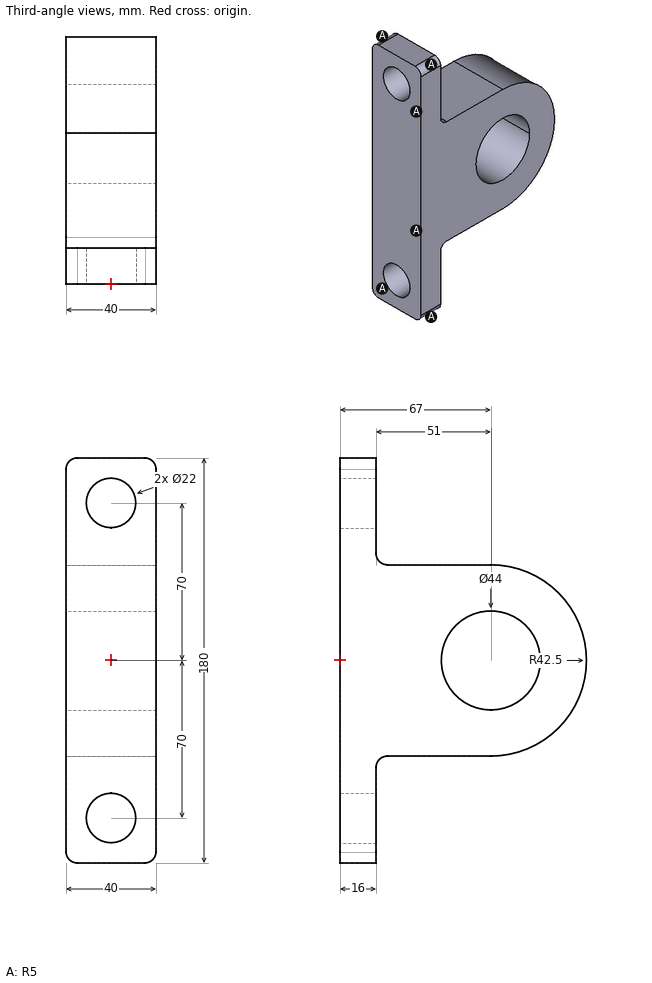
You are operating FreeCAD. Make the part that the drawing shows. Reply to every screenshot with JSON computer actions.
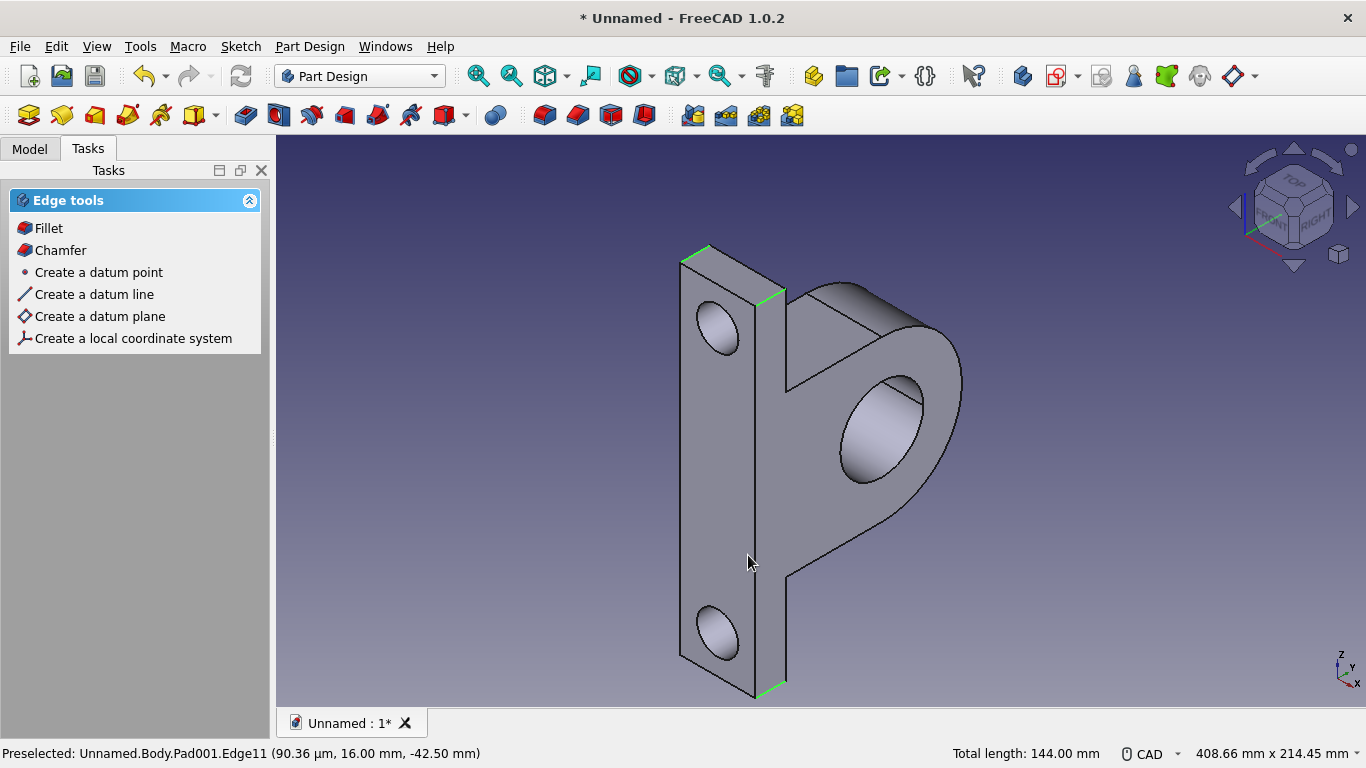
{"action": "left_click", "coordinate": [545, 116]}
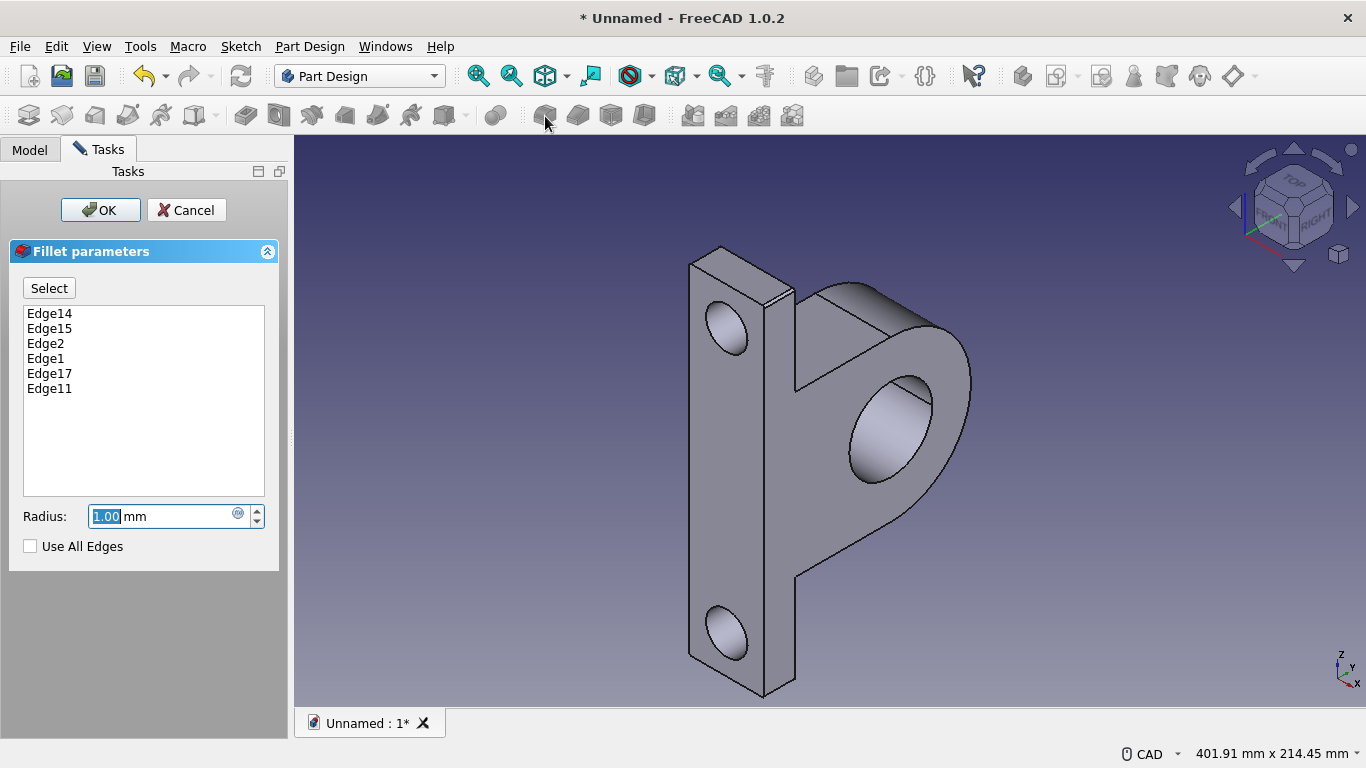
{"action": "type", "text": "5"}
{"action": "key", "text": "Tab"}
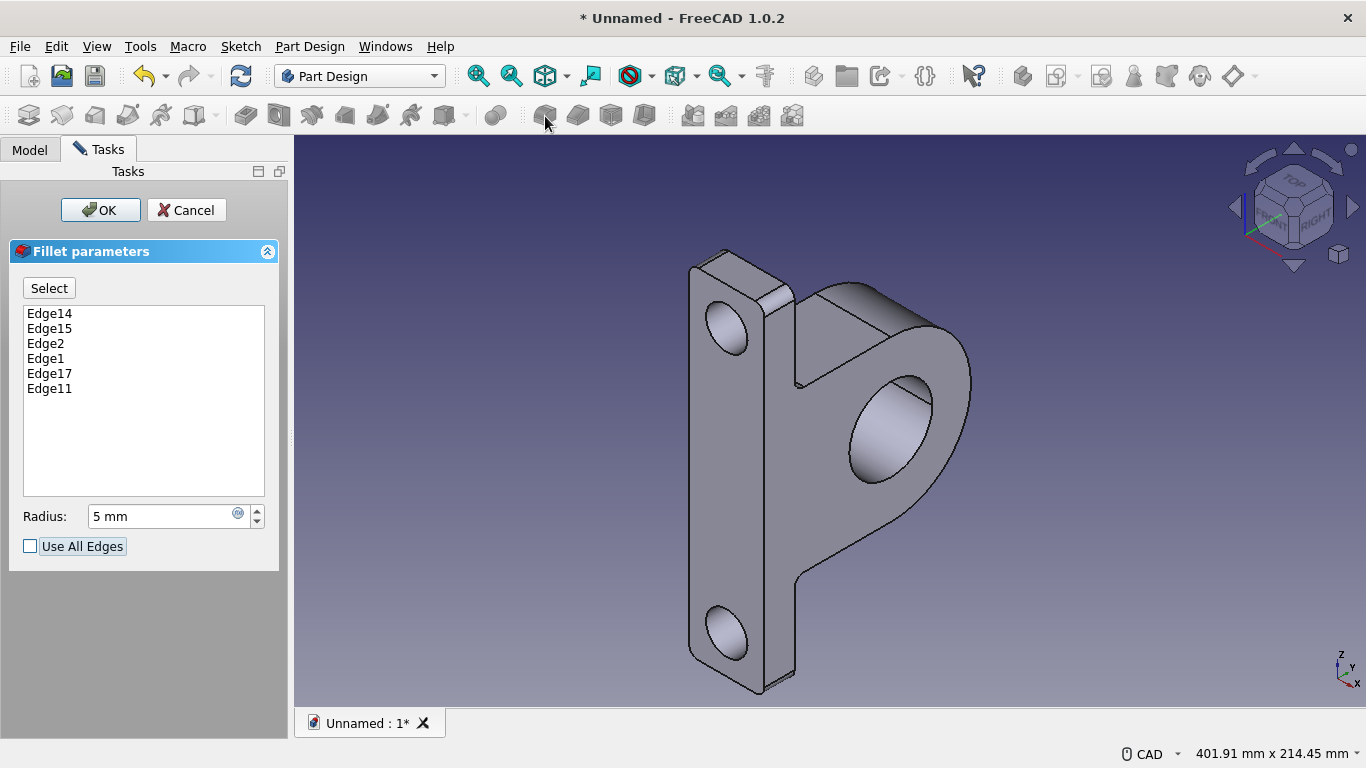
{"action": "left_click", "coordinate": [101, 210]}